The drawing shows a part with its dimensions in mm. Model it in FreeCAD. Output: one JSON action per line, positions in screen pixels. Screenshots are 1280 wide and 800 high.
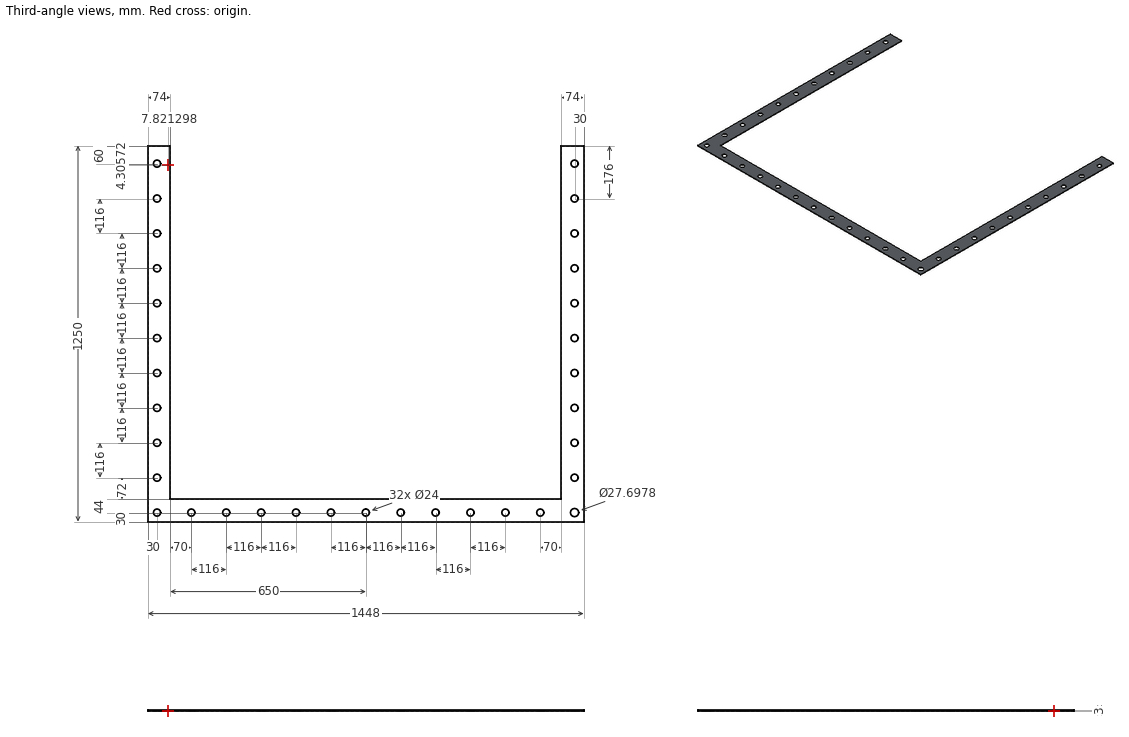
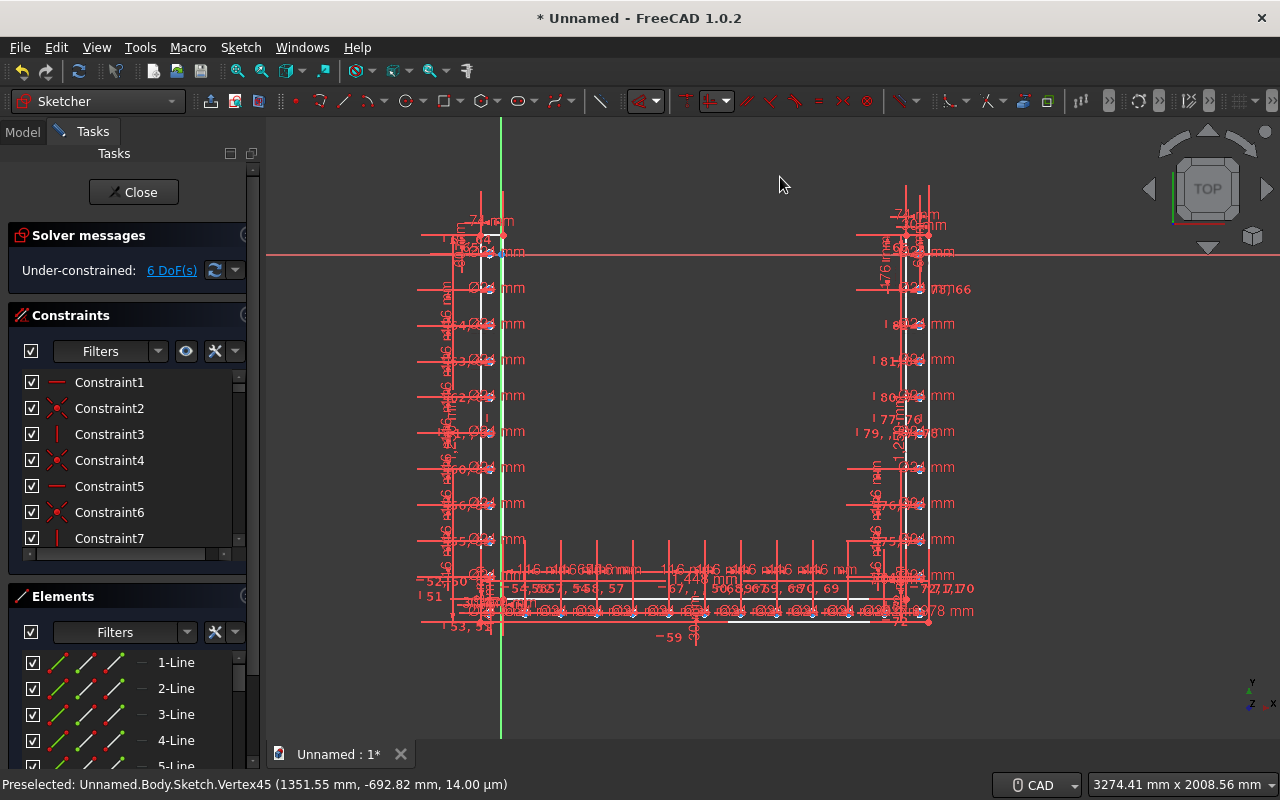
{"action": "left_click", "coordinate": [920, 469]}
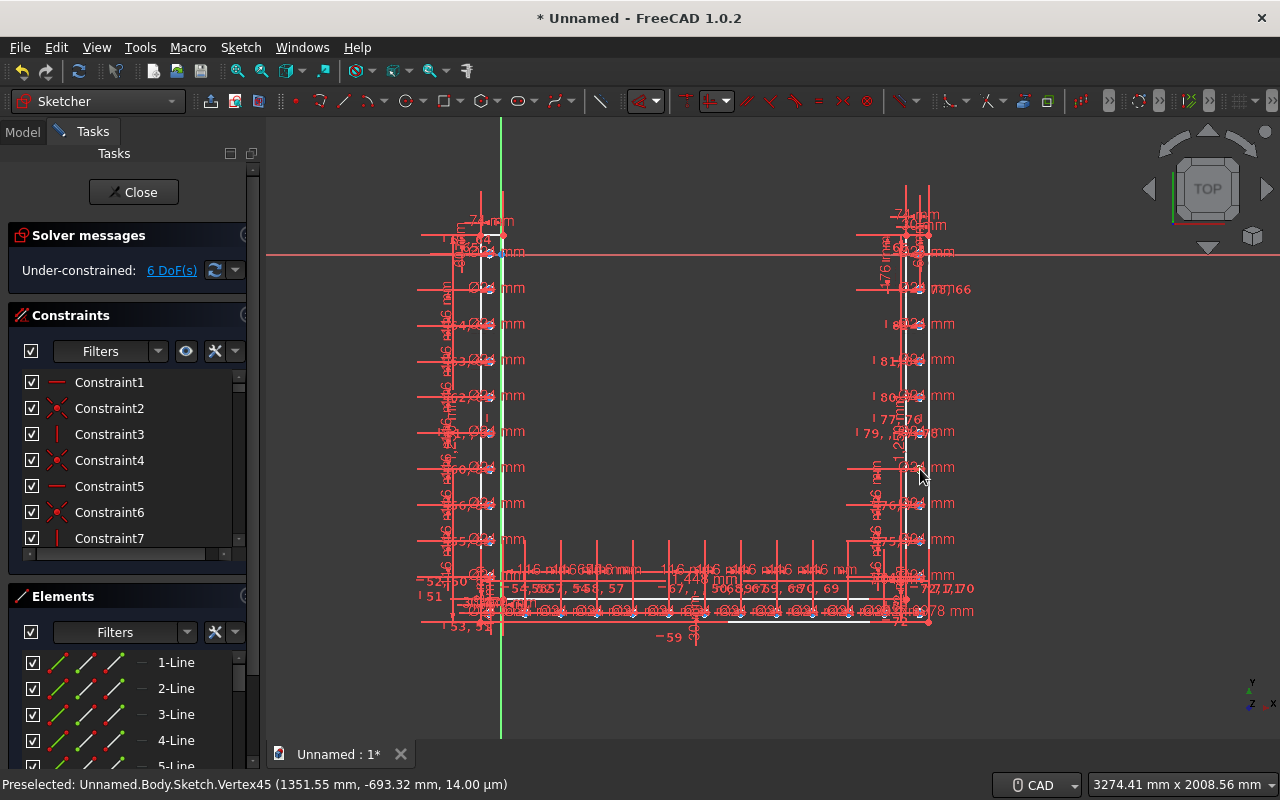
{"action": "left_click", "coordinate": [920, 433]}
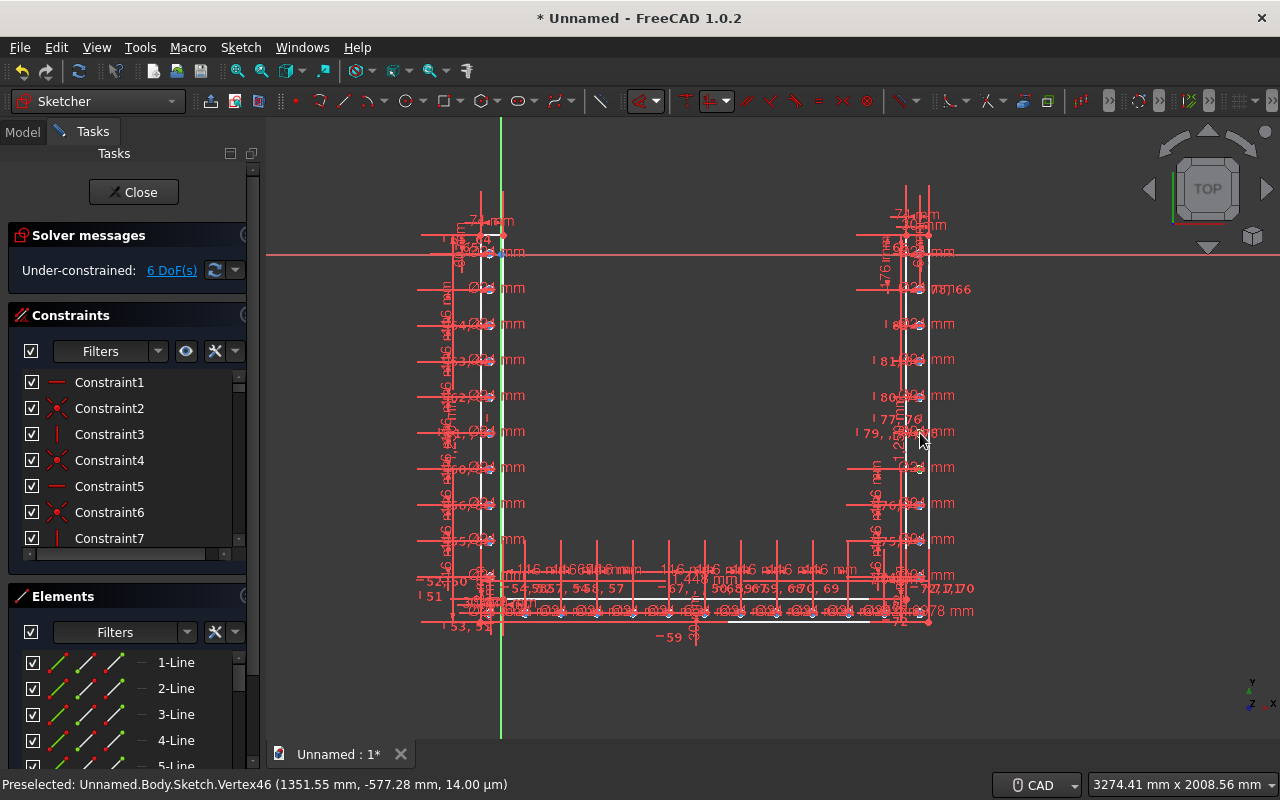
{"action": "left_click", "coordinate": [658, 102]}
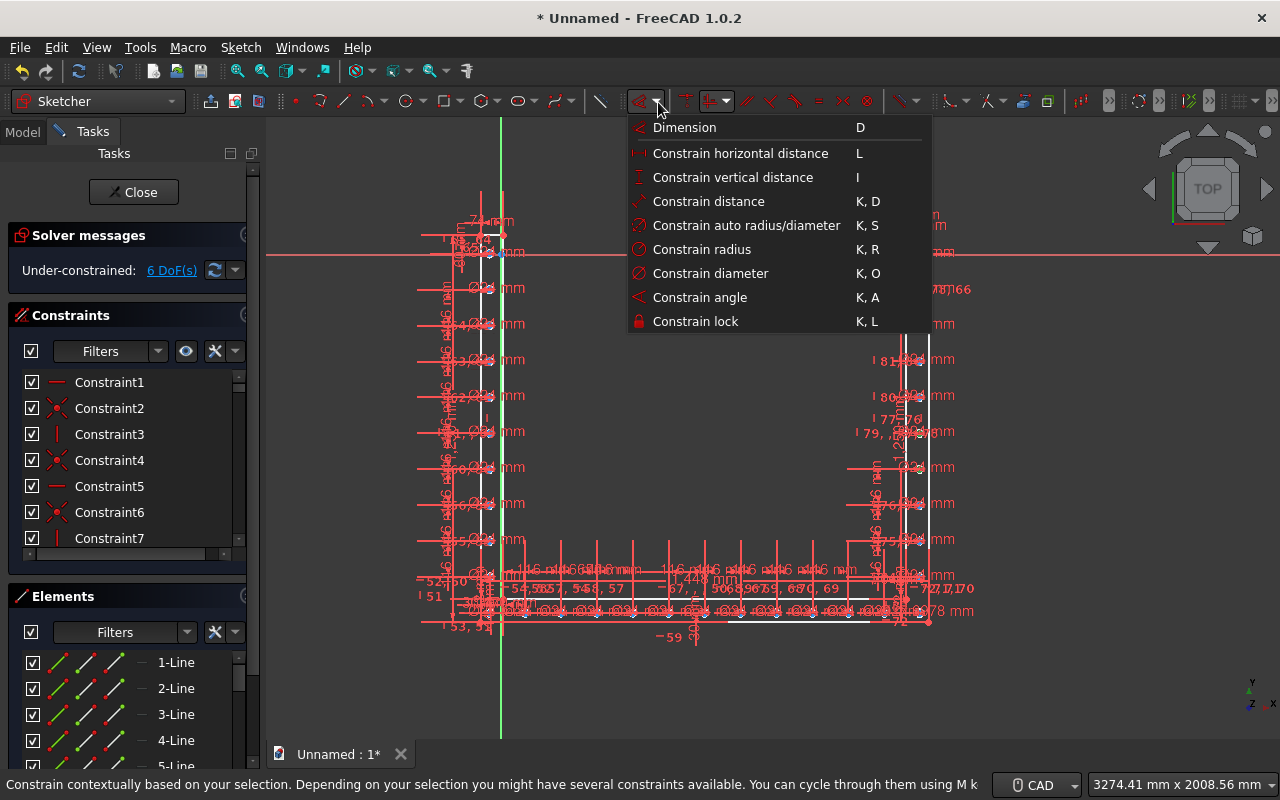
{"action": "left_click", "coordinate": [780, 177]}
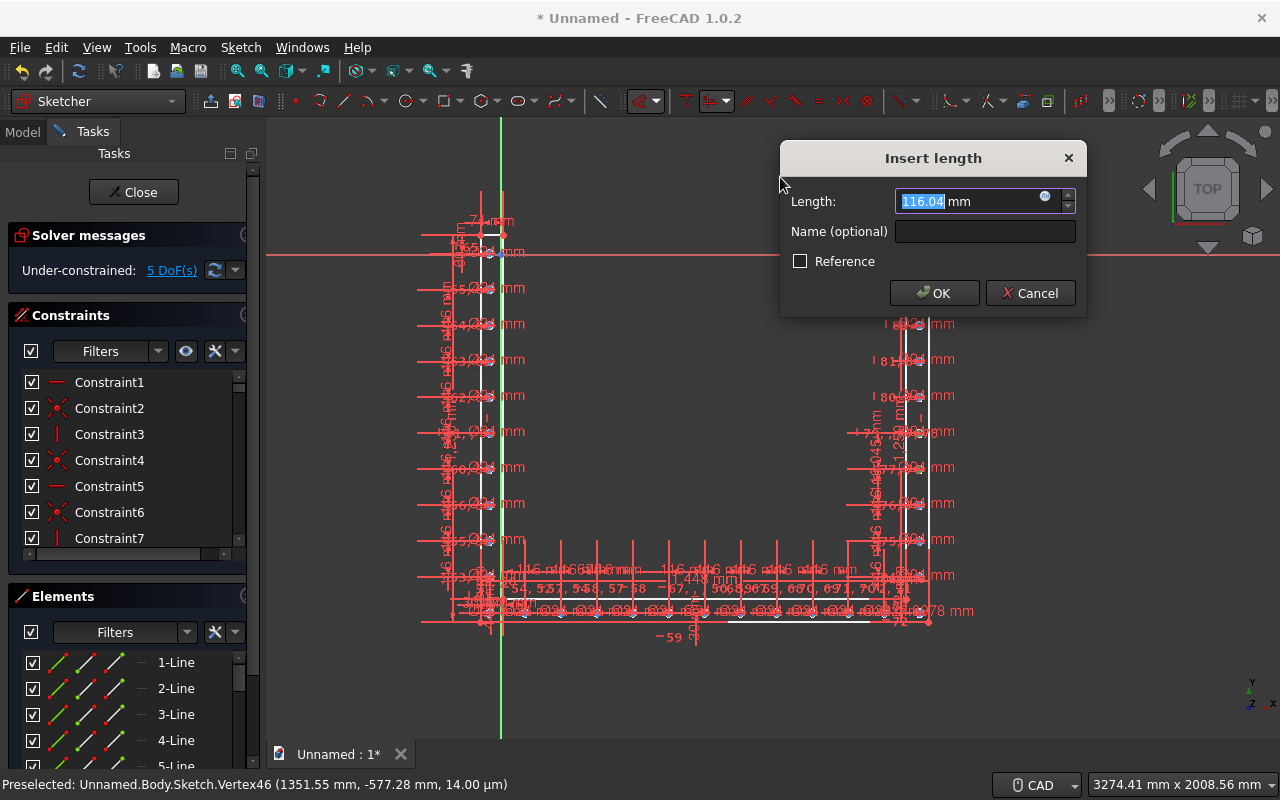
{"action": "type", "text": "116"}
{"action": "key", "text": "Return"}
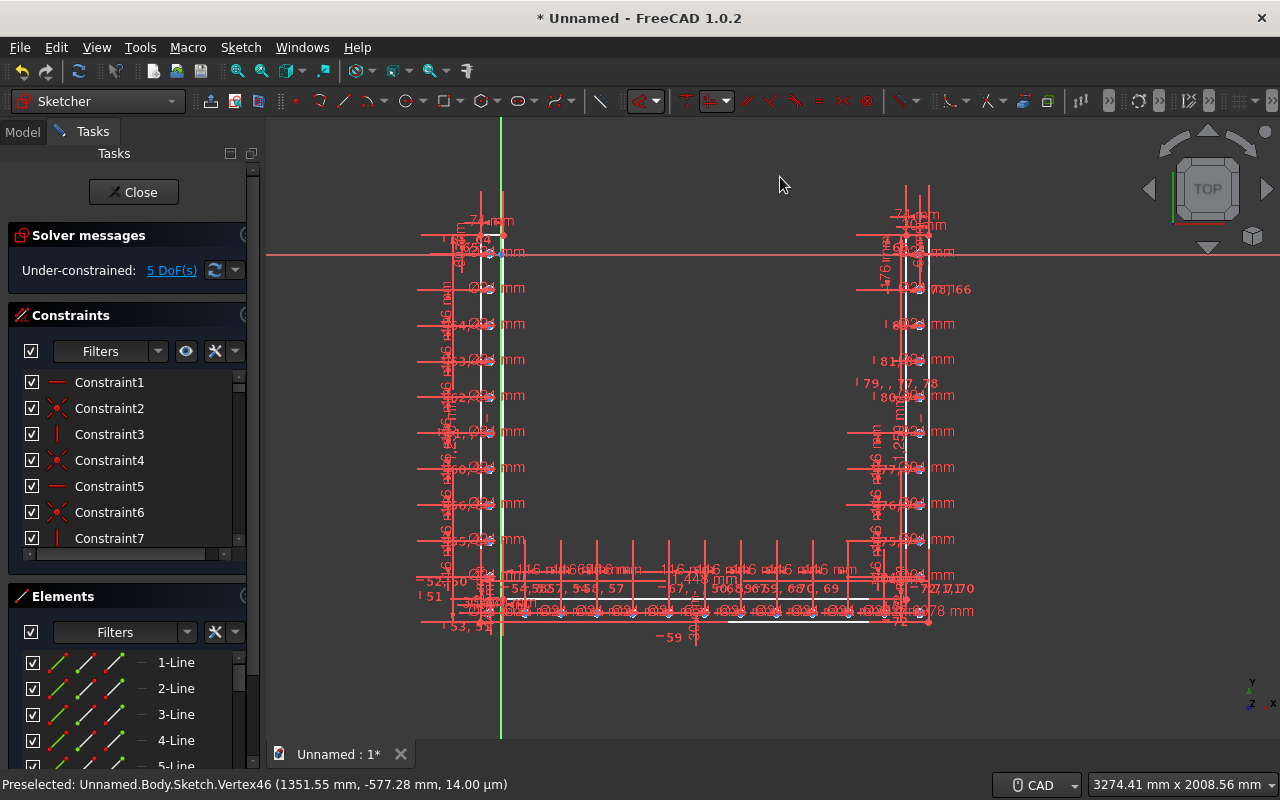
{"action": "left_click", "coordinate": [920, 433]}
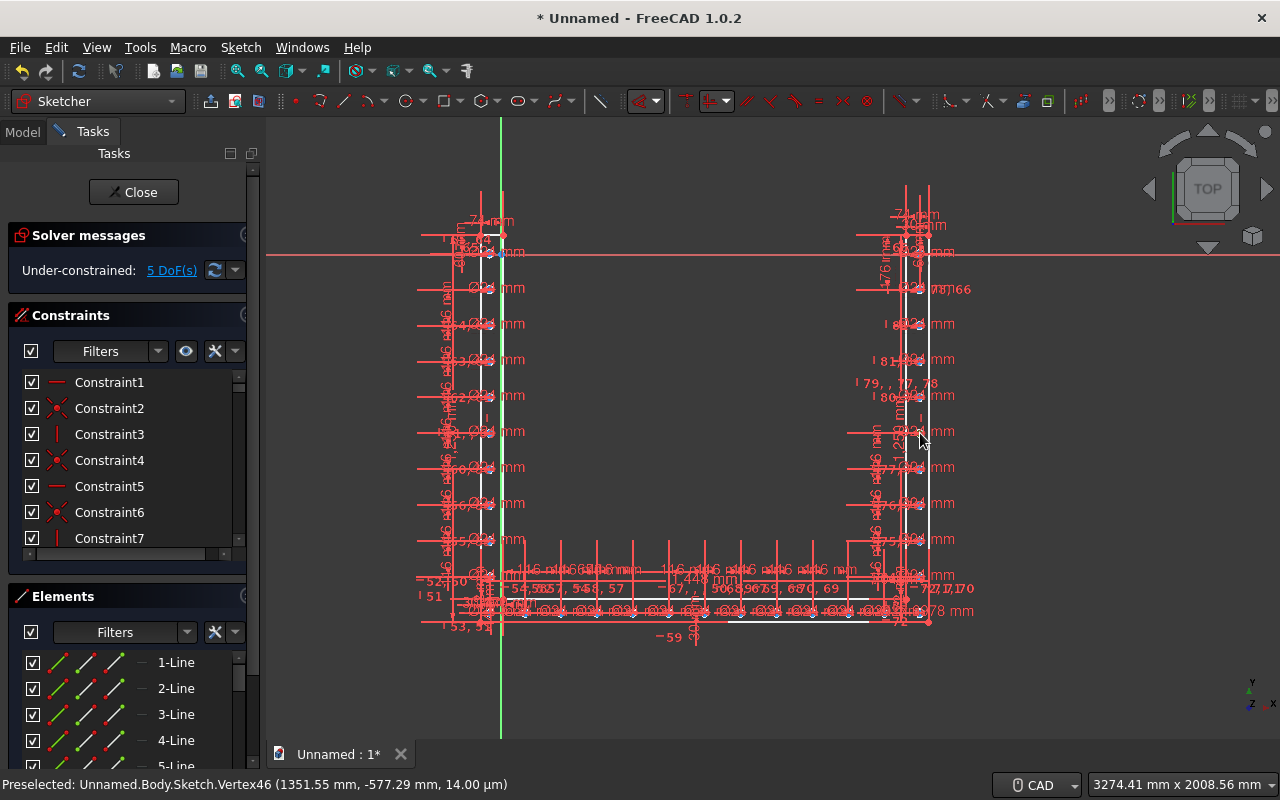
{"action": "left_click", "coordinate": [920, 397]}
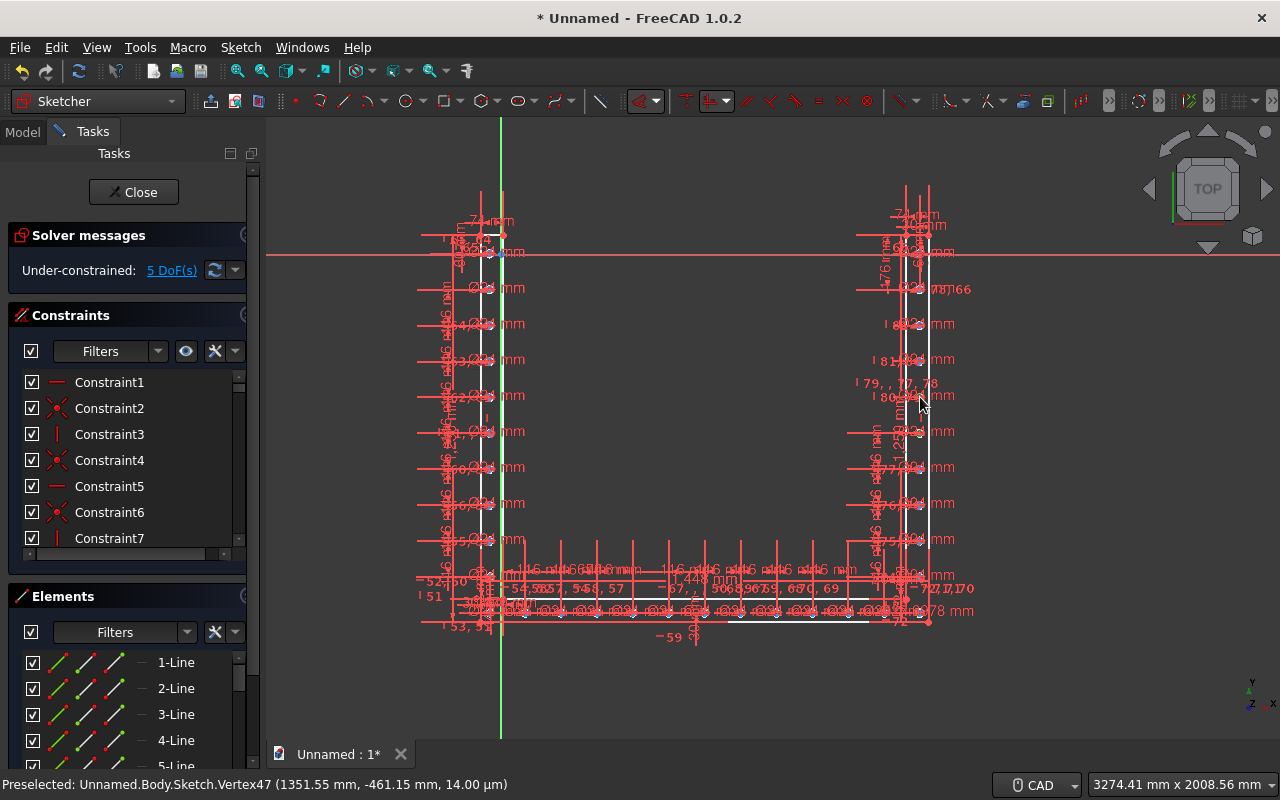
{"action": "key", "text": "i"}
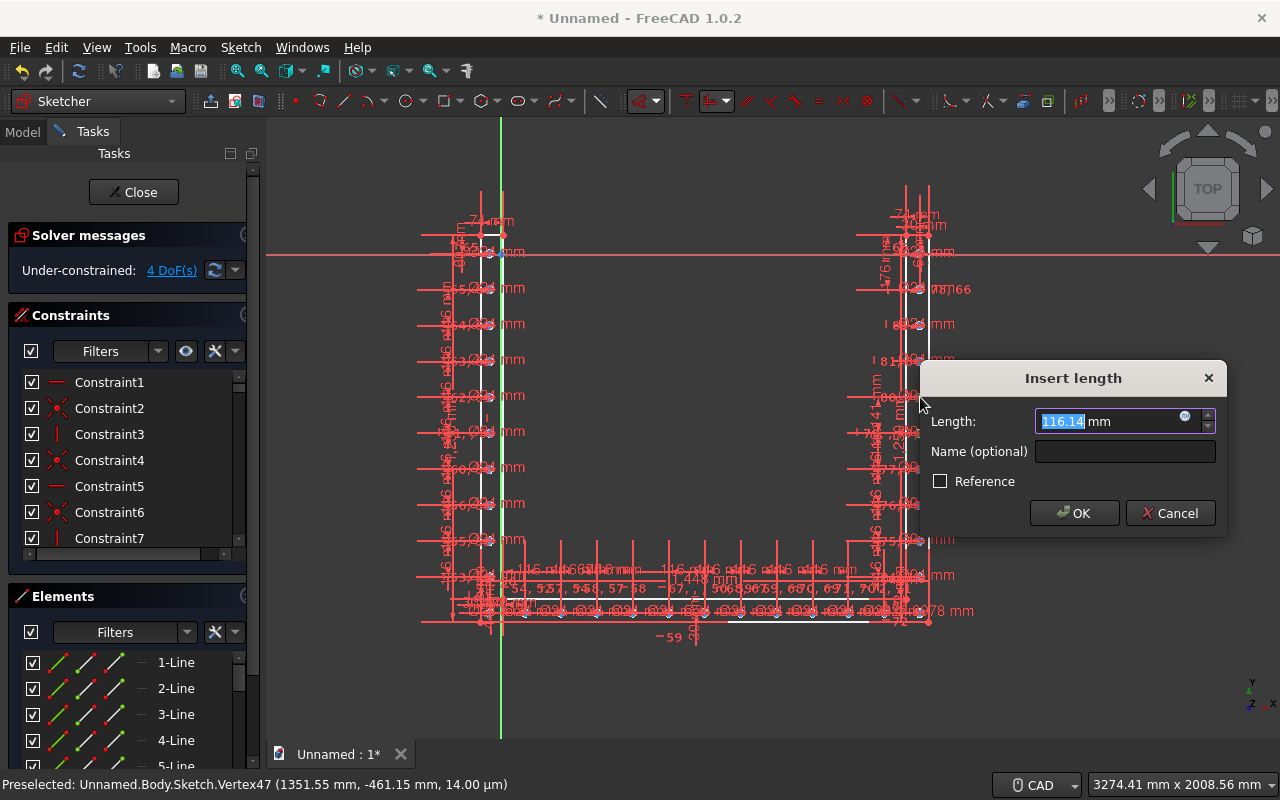
{"action": "type", "text": "116"}
{"action": "key", "text": "Return"}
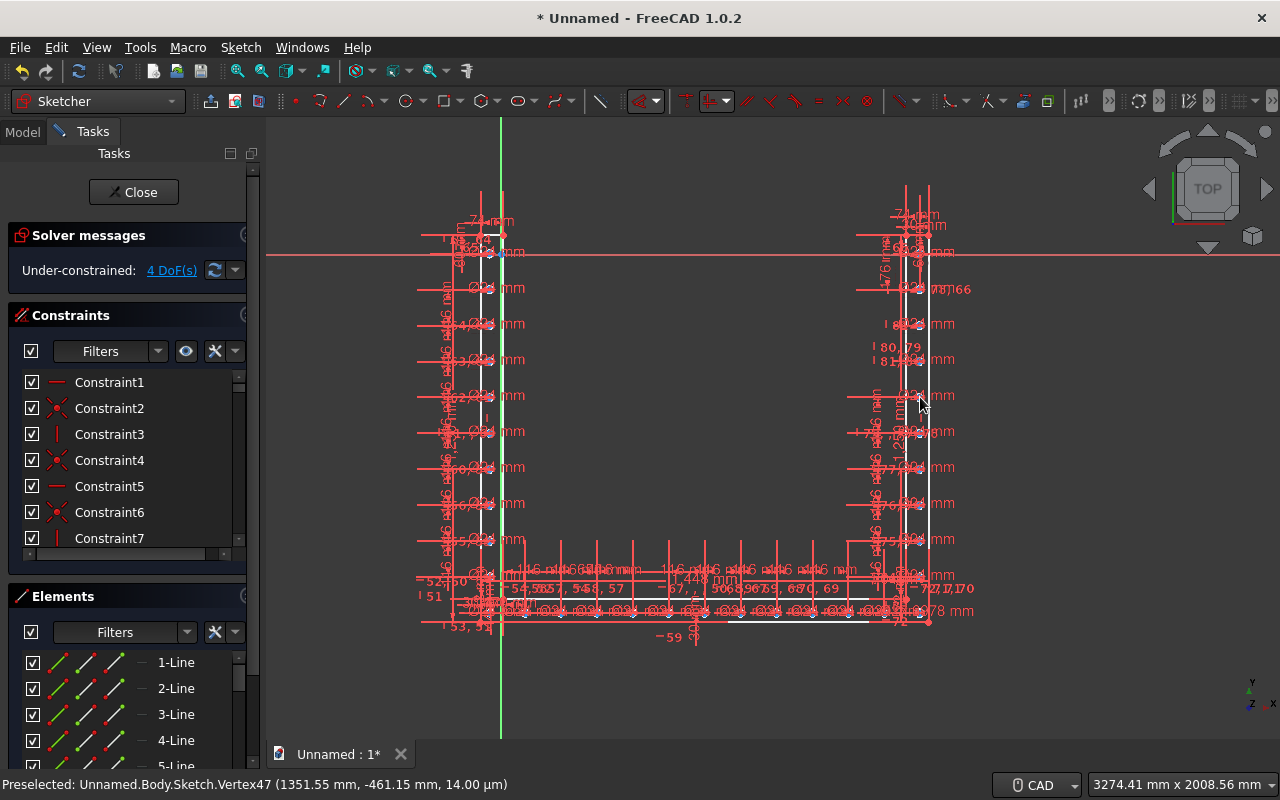
{"action": "left_click", "coordinate": [920, 397]}